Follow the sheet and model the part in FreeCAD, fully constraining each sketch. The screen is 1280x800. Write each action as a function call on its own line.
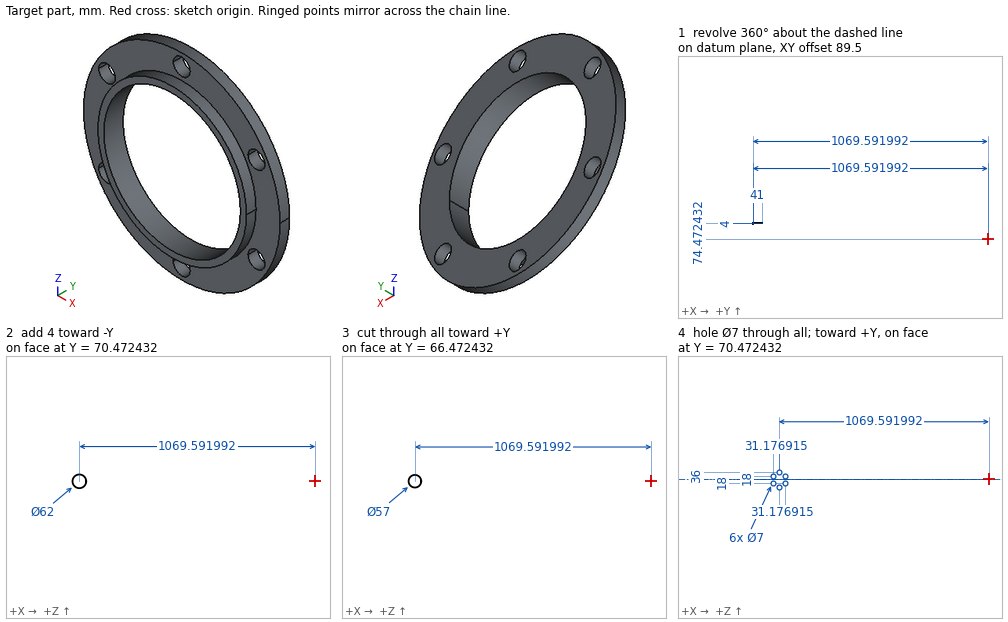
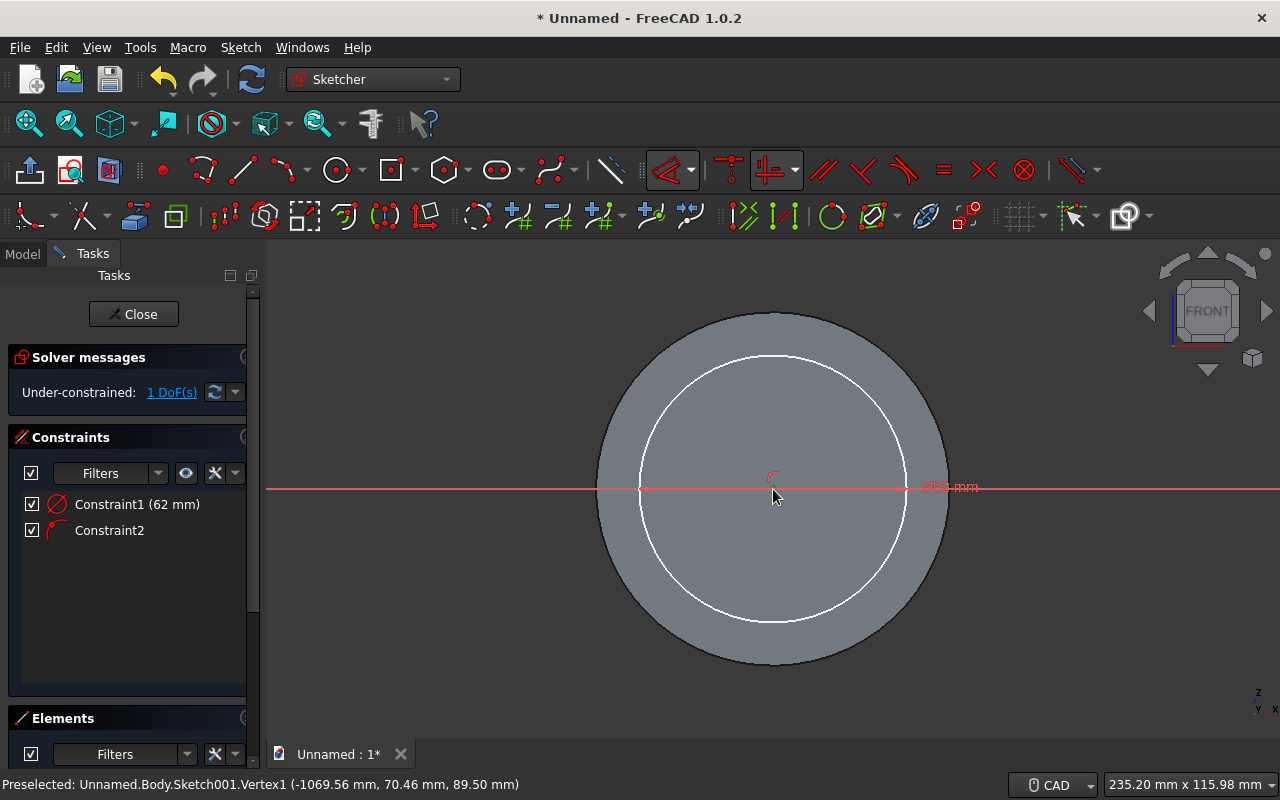
click(694, 170)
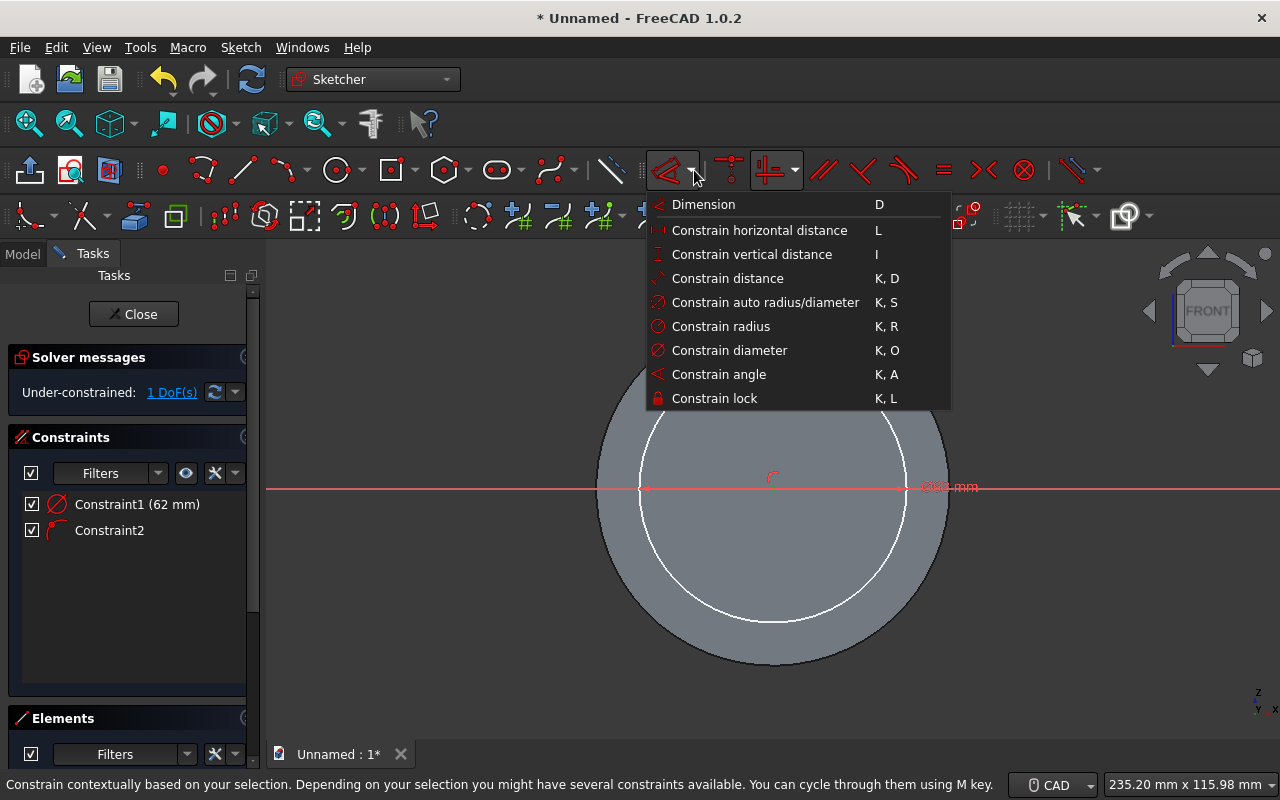
click(799, 230)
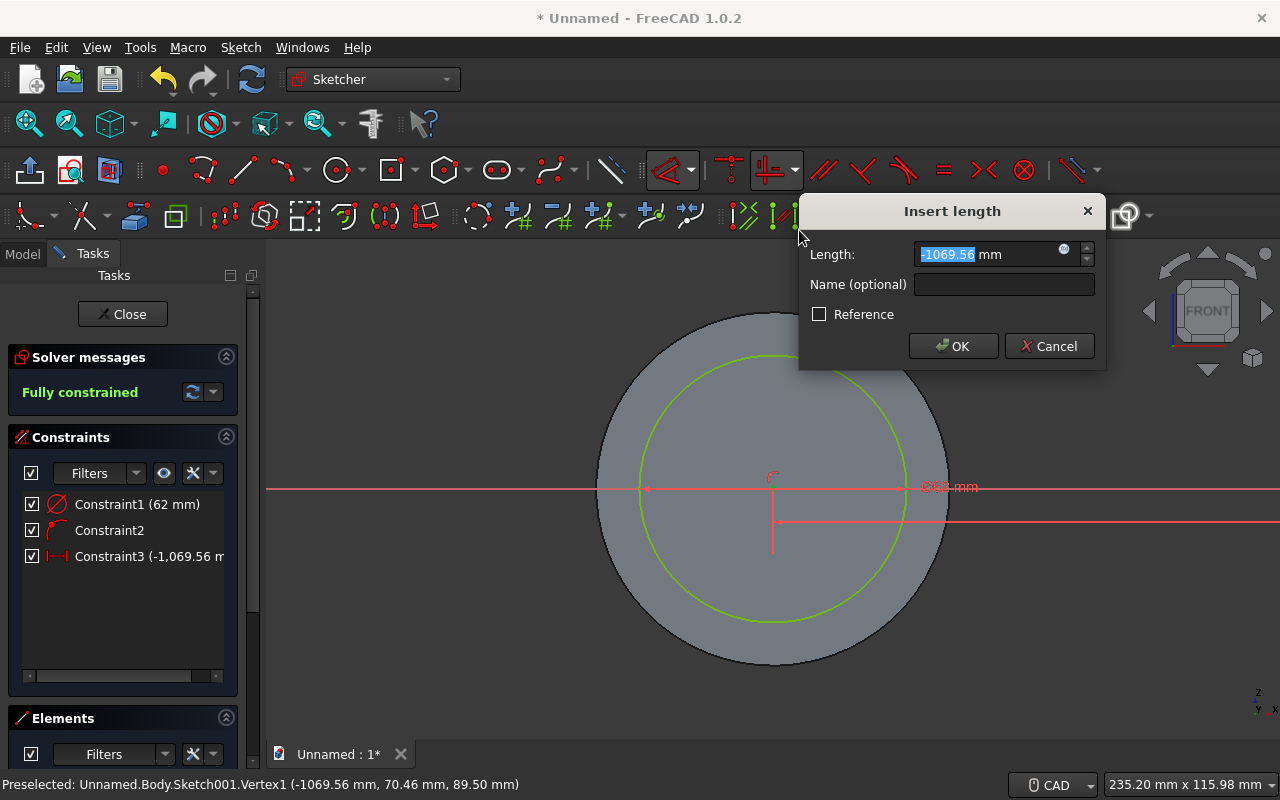
text(-1069.591992)
key(Return)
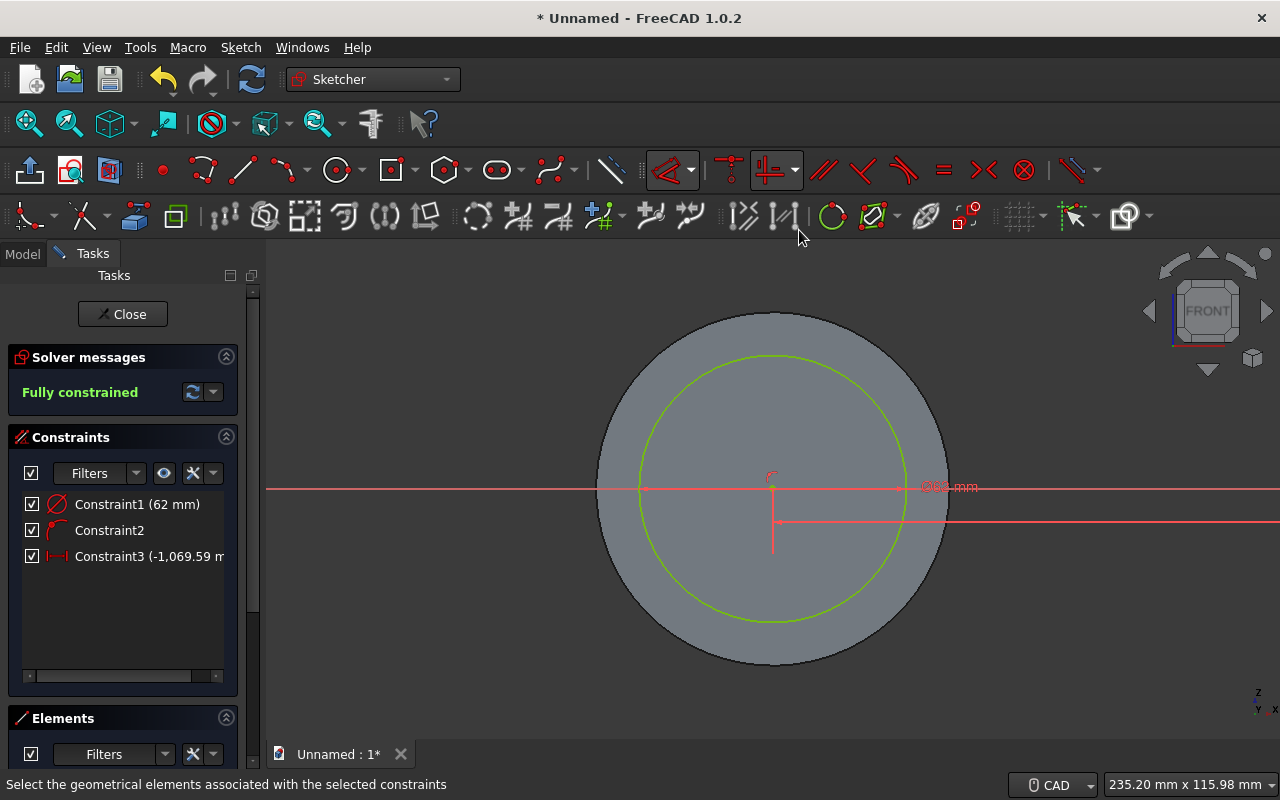
click(123, 314)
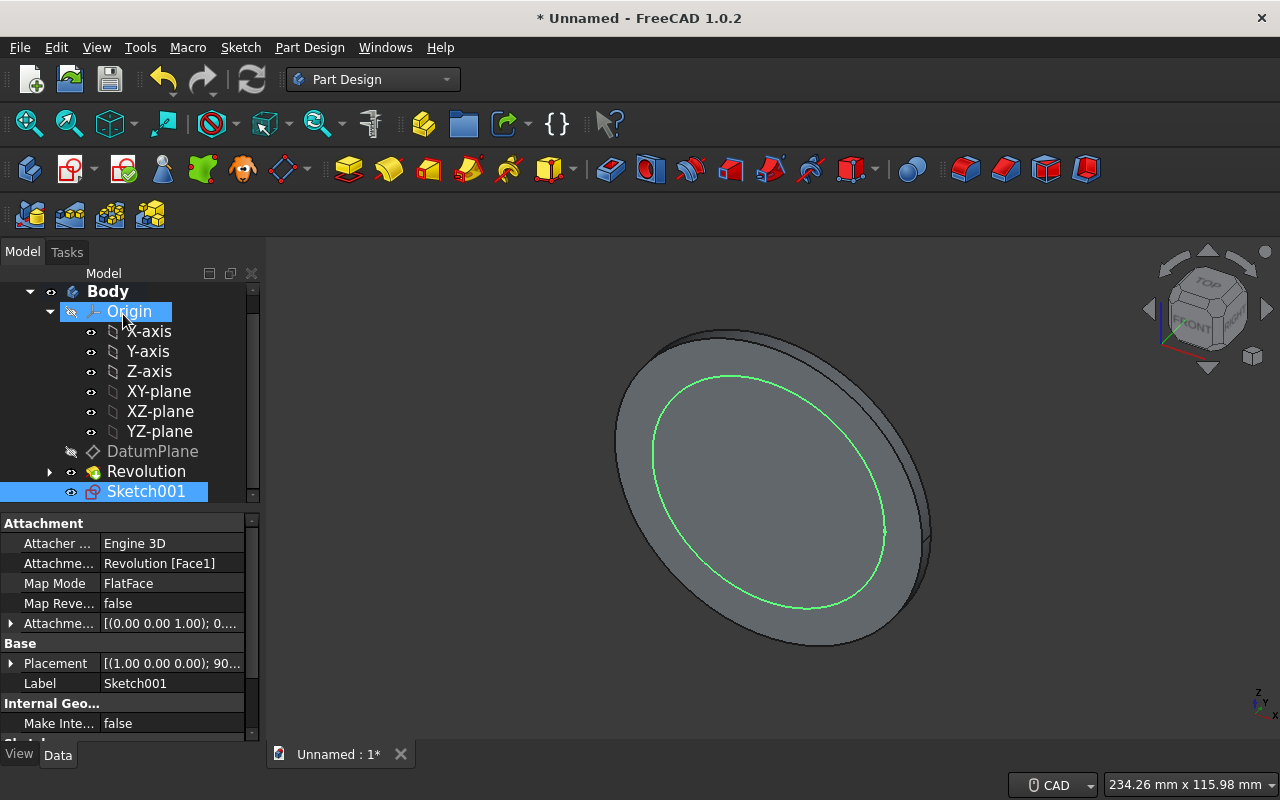
click(350, 170)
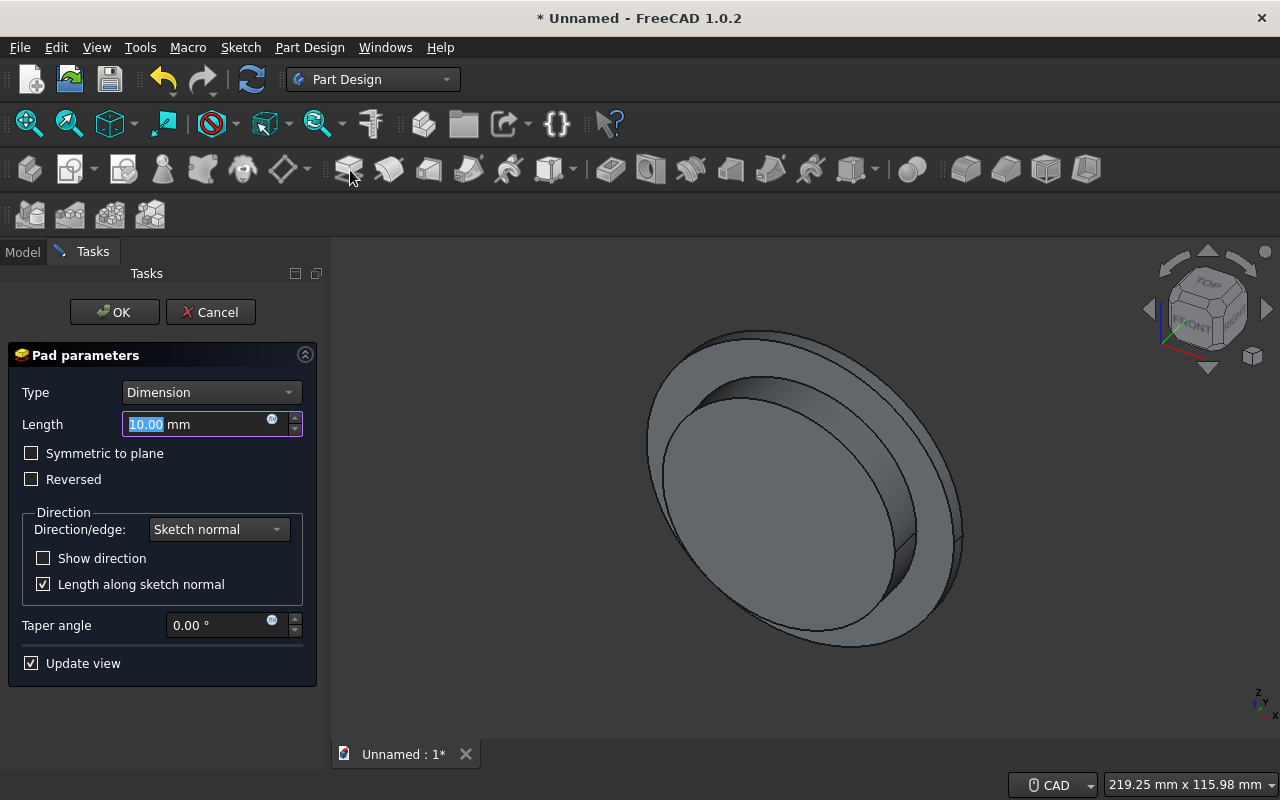
text(4)
key(Tab)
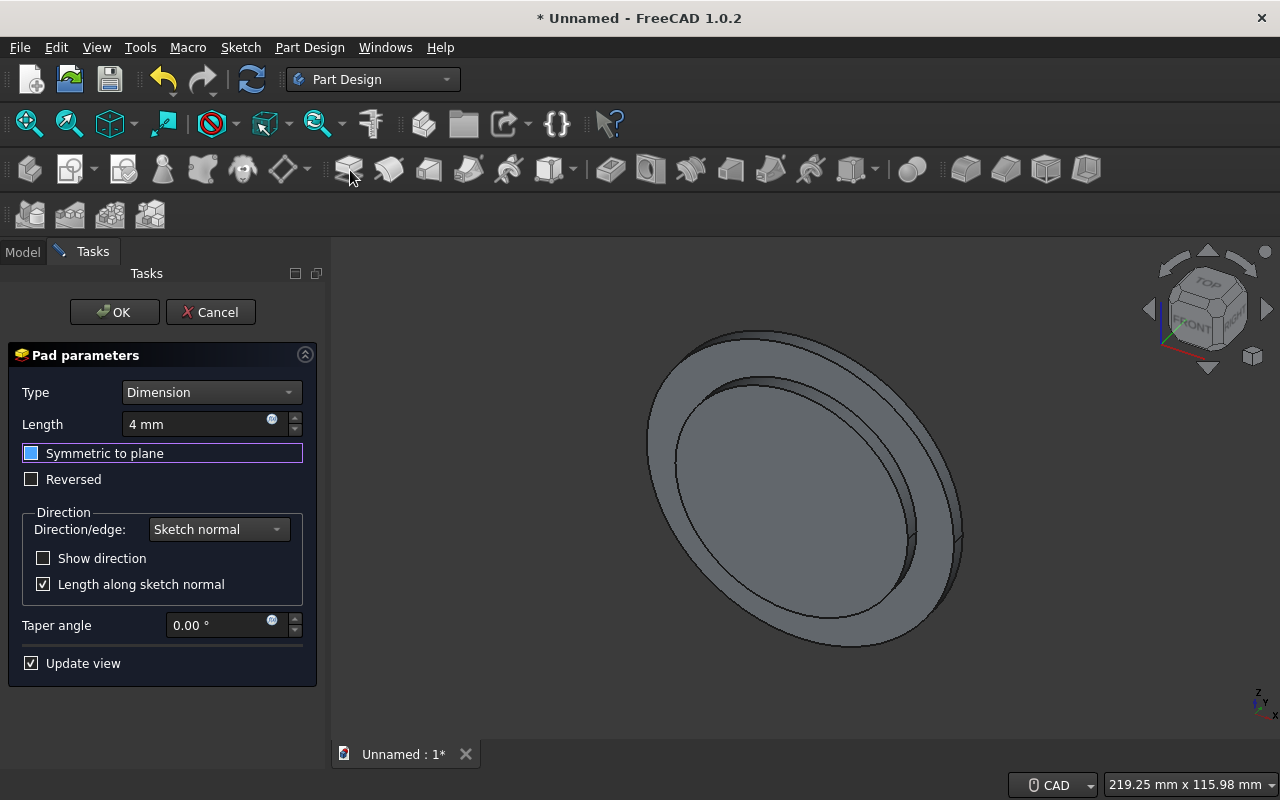
click(115, 312)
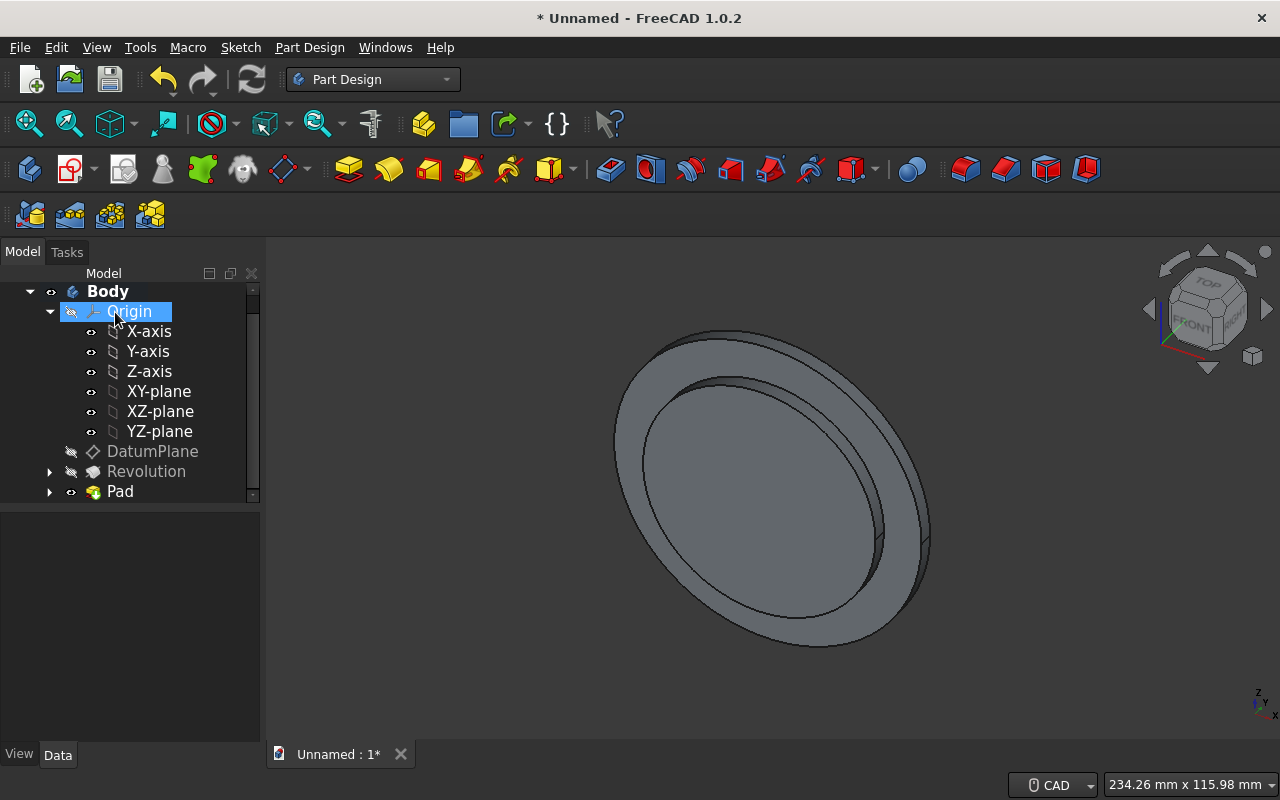
click(759, 501)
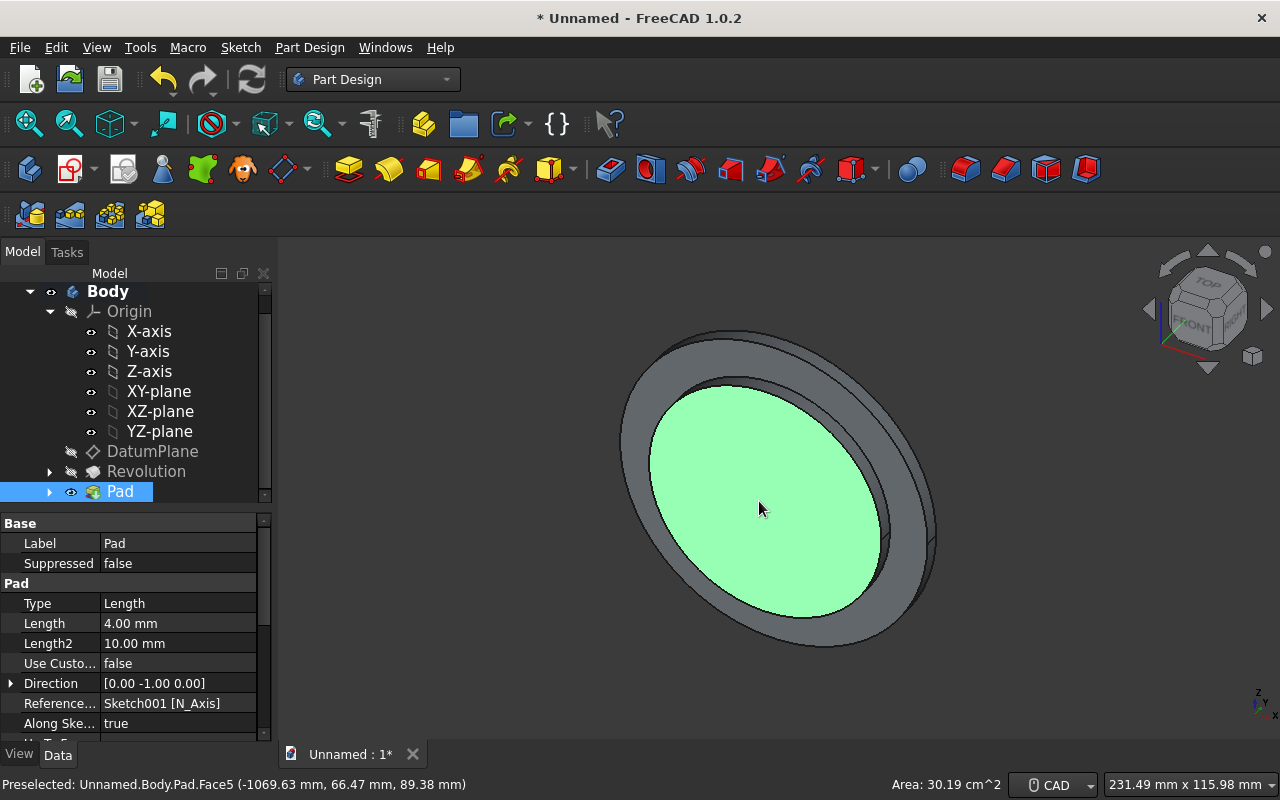
click(70, 170)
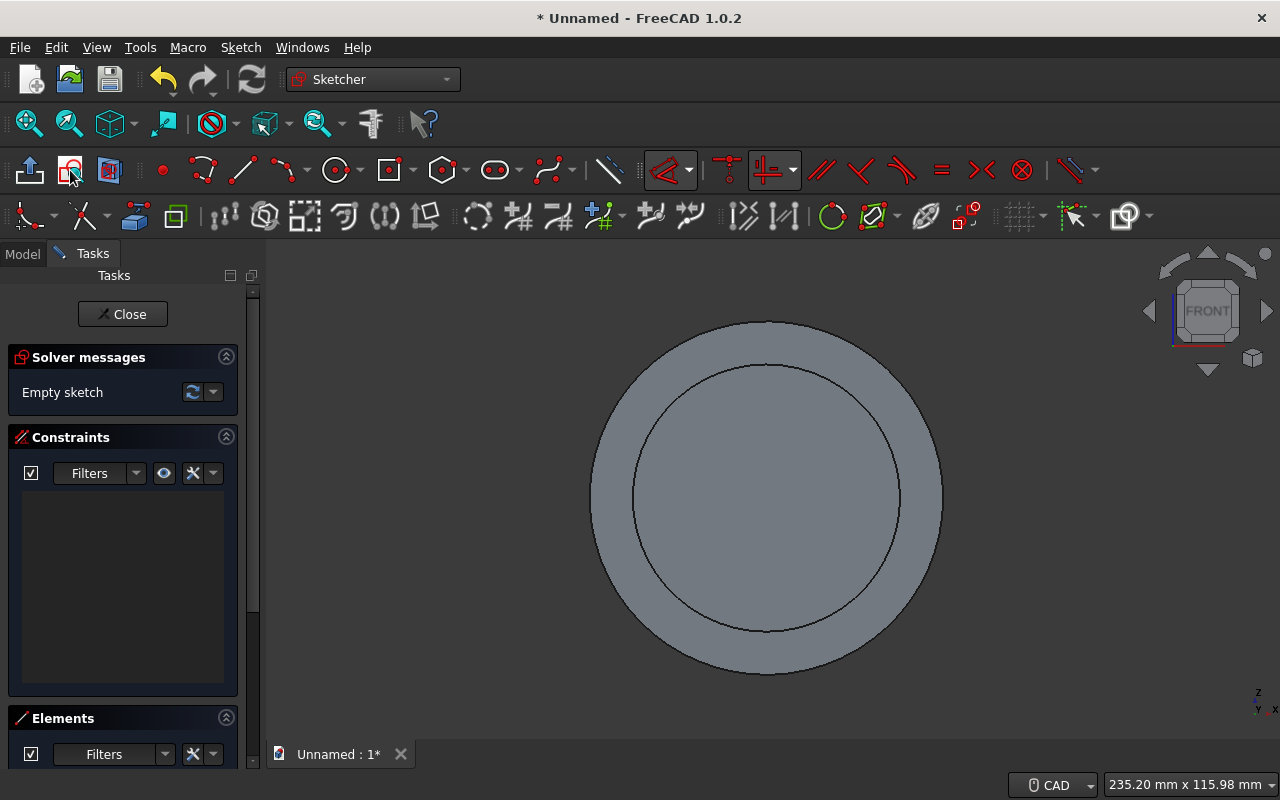
click(336, 170)